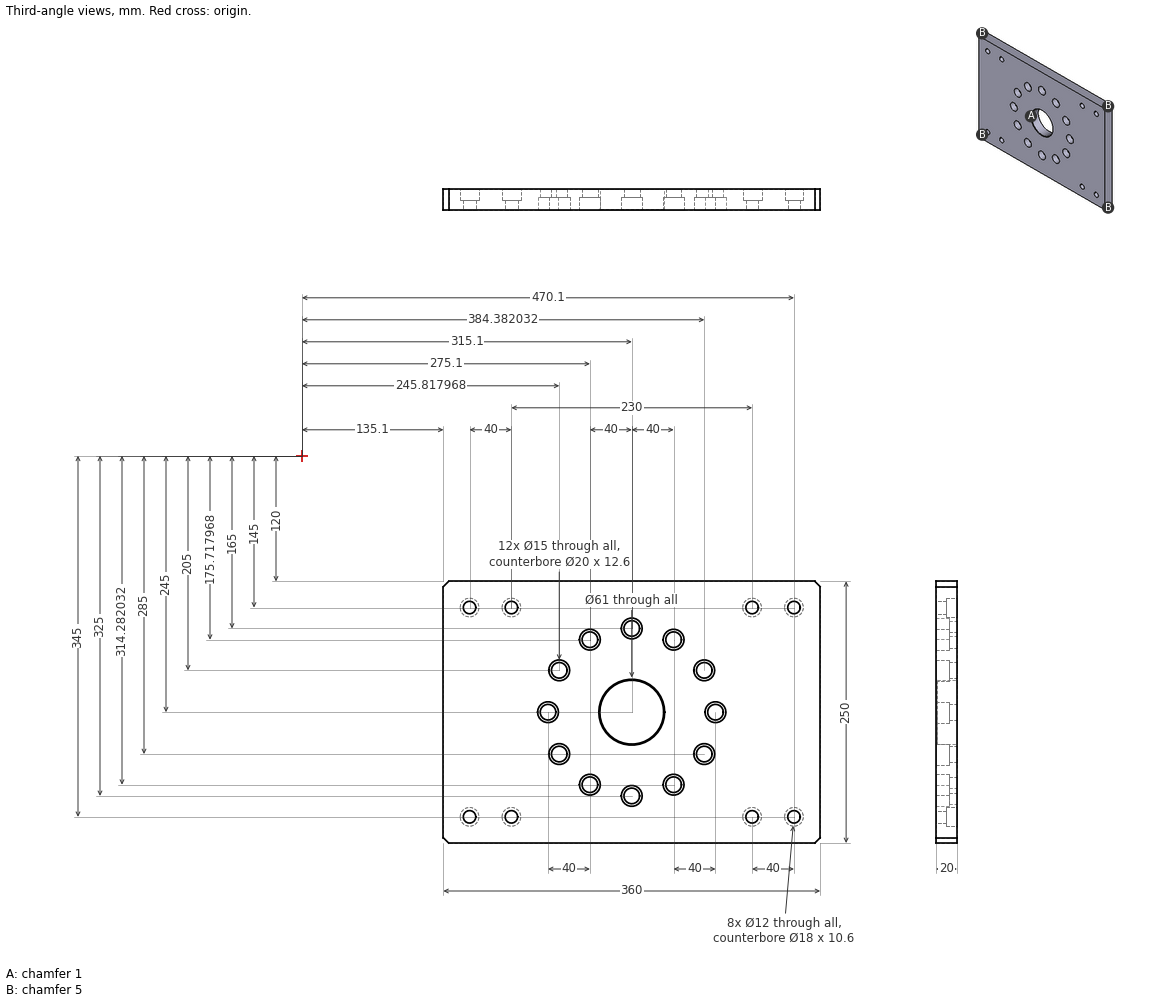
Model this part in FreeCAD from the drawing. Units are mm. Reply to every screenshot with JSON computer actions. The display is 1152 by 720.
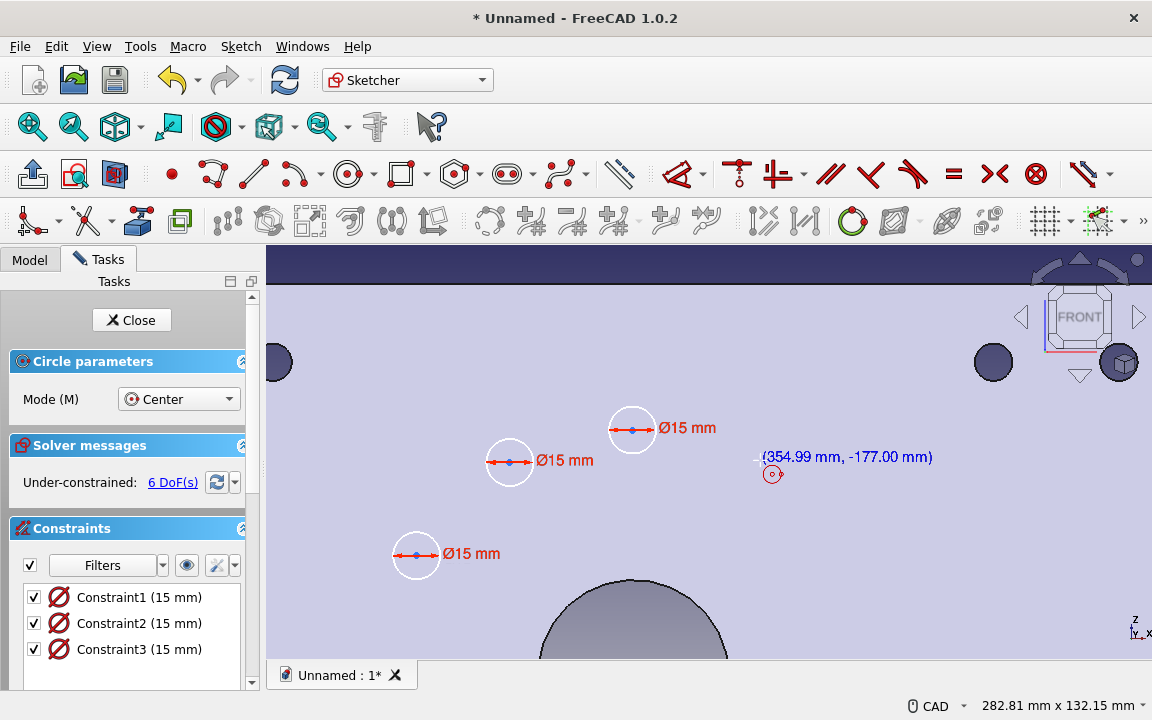
{"action": "scroll", "coordinate": [760, 460], "scroll_direction": "down", "scroll_amount": 7}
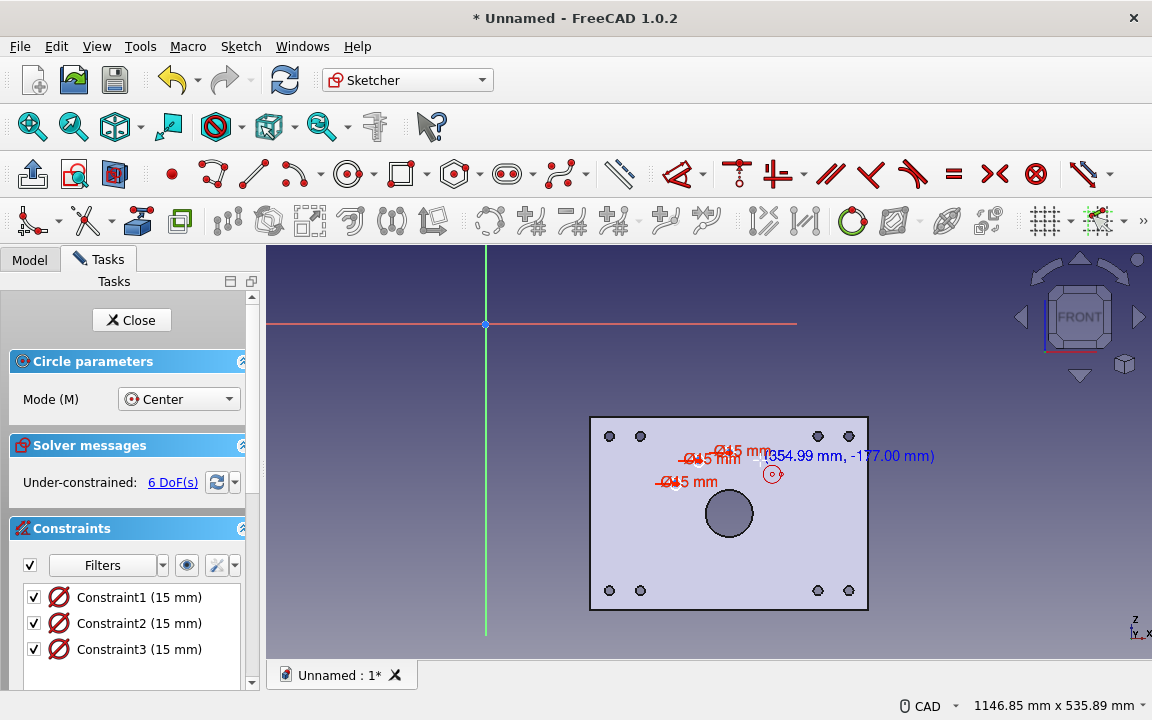
{"action": "left_click", "coordinate": [760, 460]}
{"action": "mouse_move", "coordinate": [764, 456]}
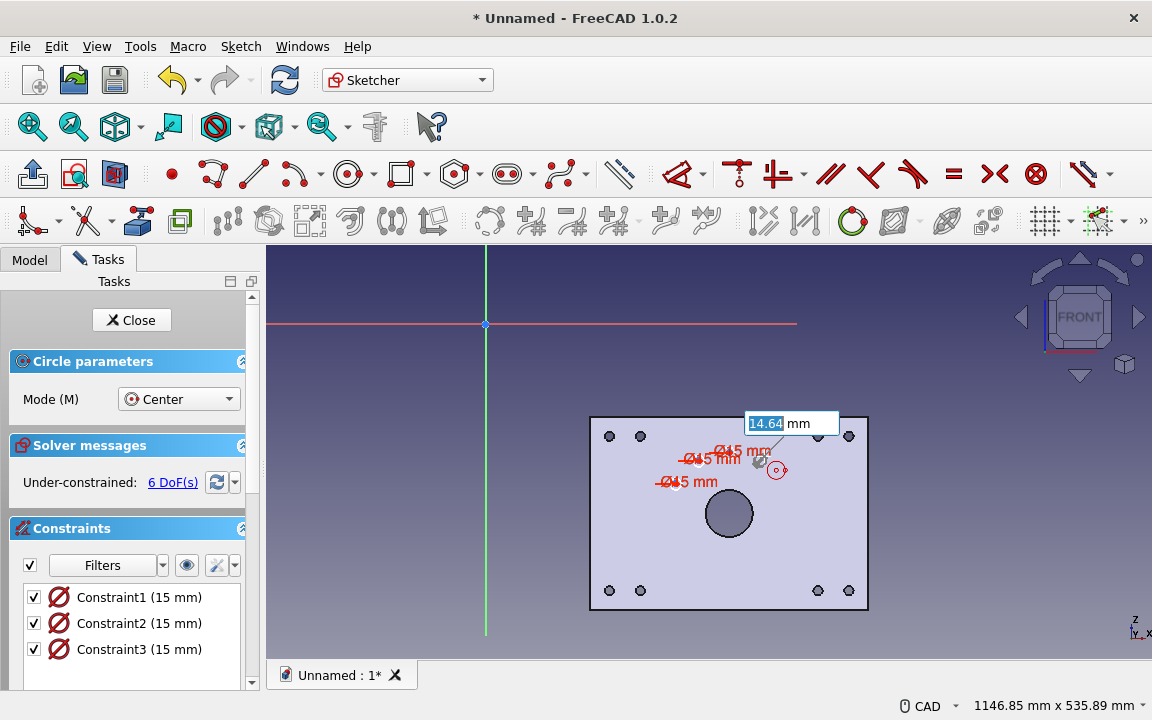
{"action": "type", "text": "15"}
{"action": "key", "text": "Return"}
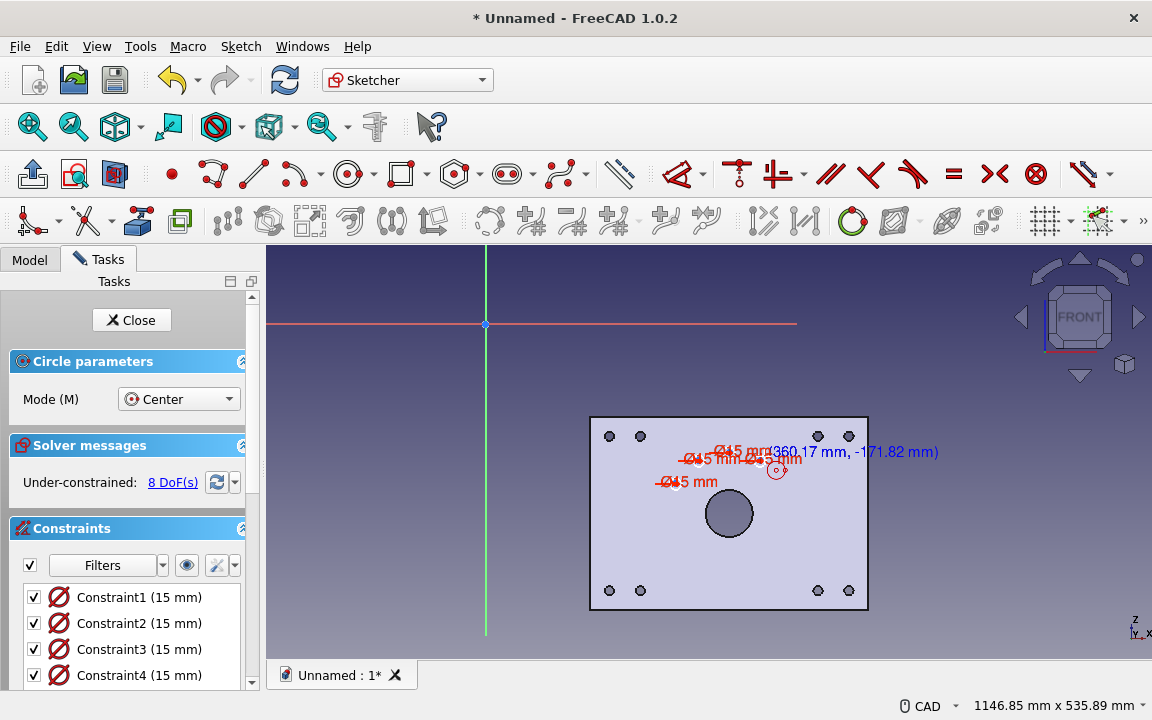
{"action": "scroll", "coordinate": [783, 483], "scroll_direction": "up", "scroll_amount": 7}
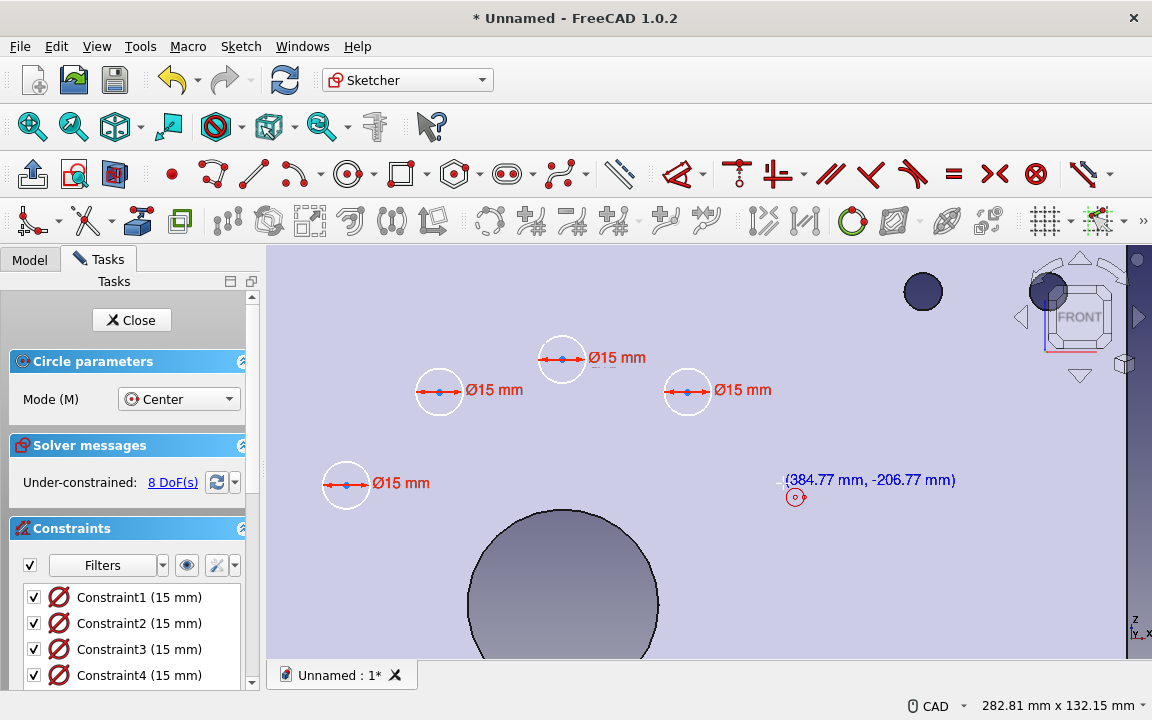
{"action": "scroll", "coordinate": [783, 483], "scroll_direction": "down", "scroll_amount": 7}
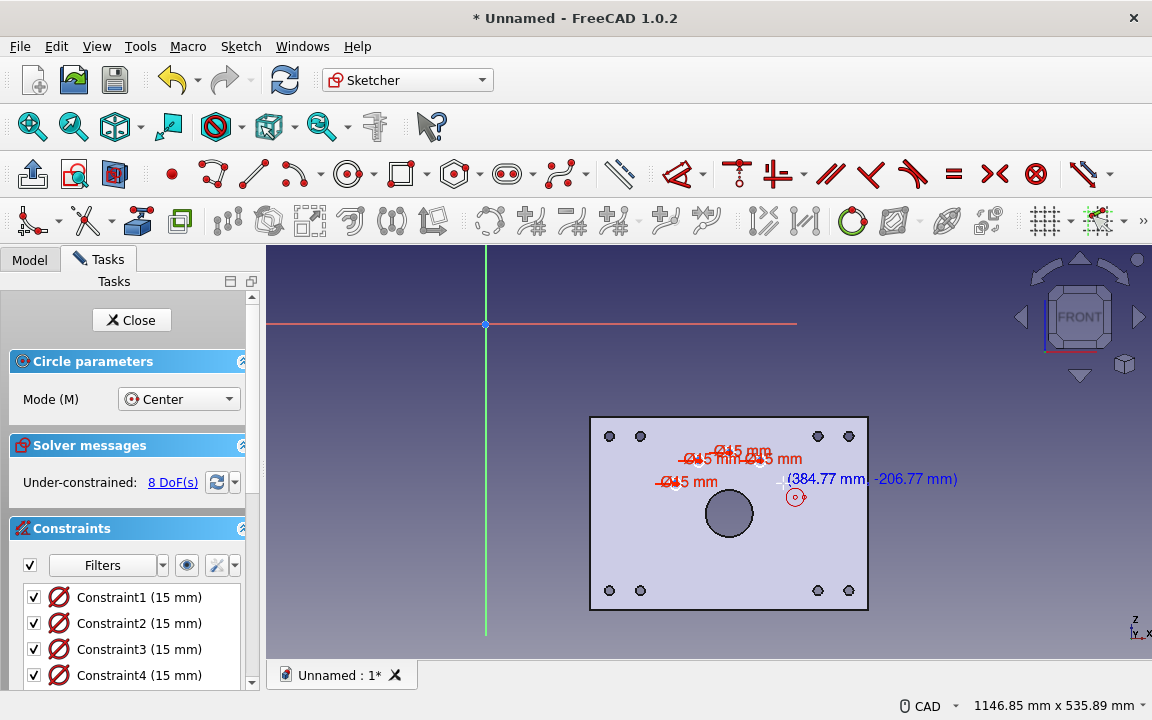
{"action": "left_click", "coordinate": [783, 483]}
{"action": "mouse_move", "coordinate": [787, 479]}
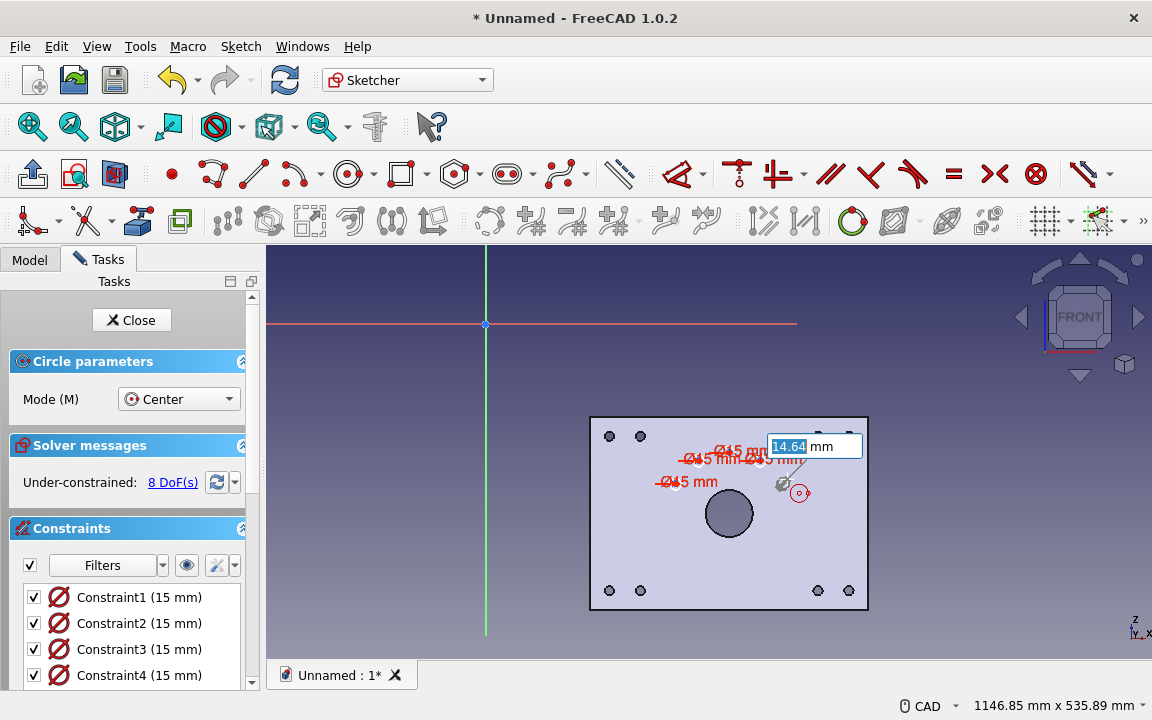
{"action": "type", "text": "15"}
{"action": "key", "text": "Return"}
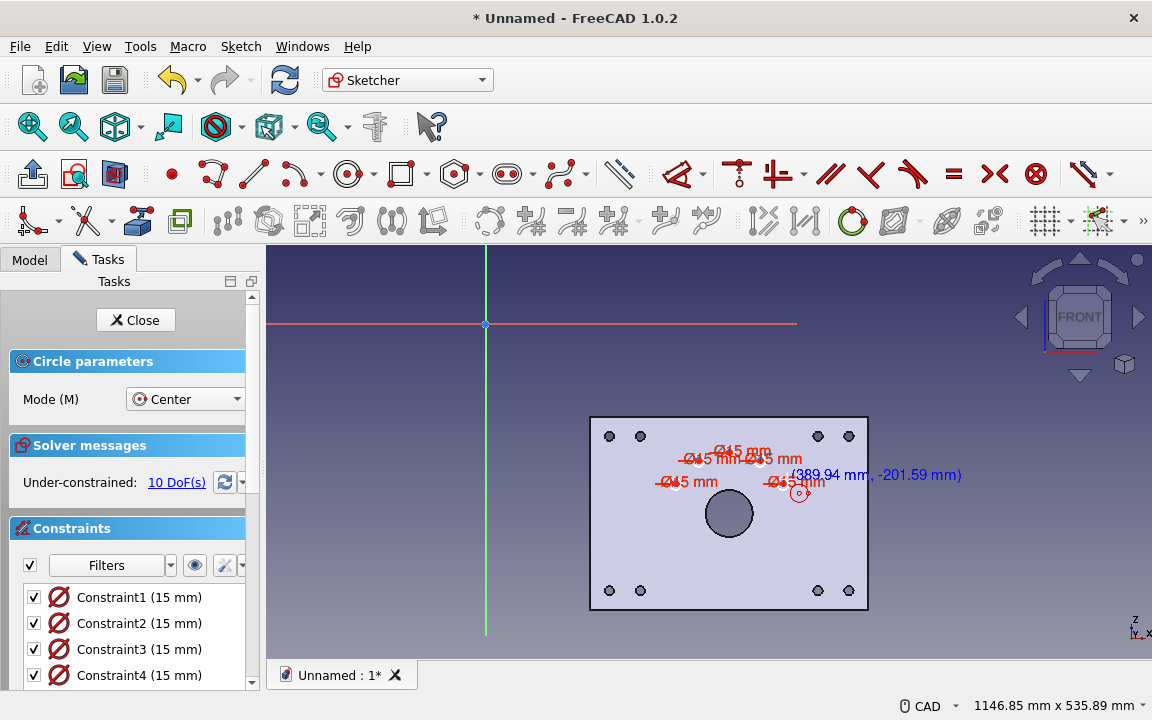
{"action": "scroll", "coordinate": [791, 514], "scroll_direction": "up", "scroll_amount": 7}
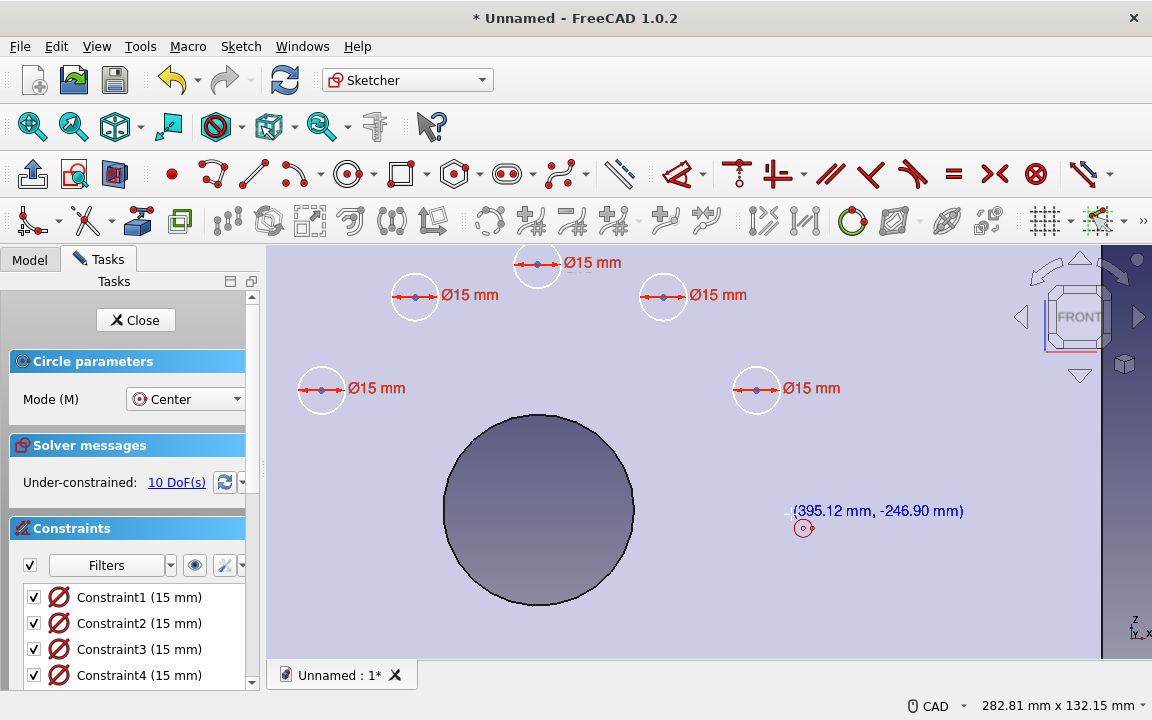
{"action": "scroll", "coordinate": [791, 514], "scroll_direction": "down", "scroll_amount": 7}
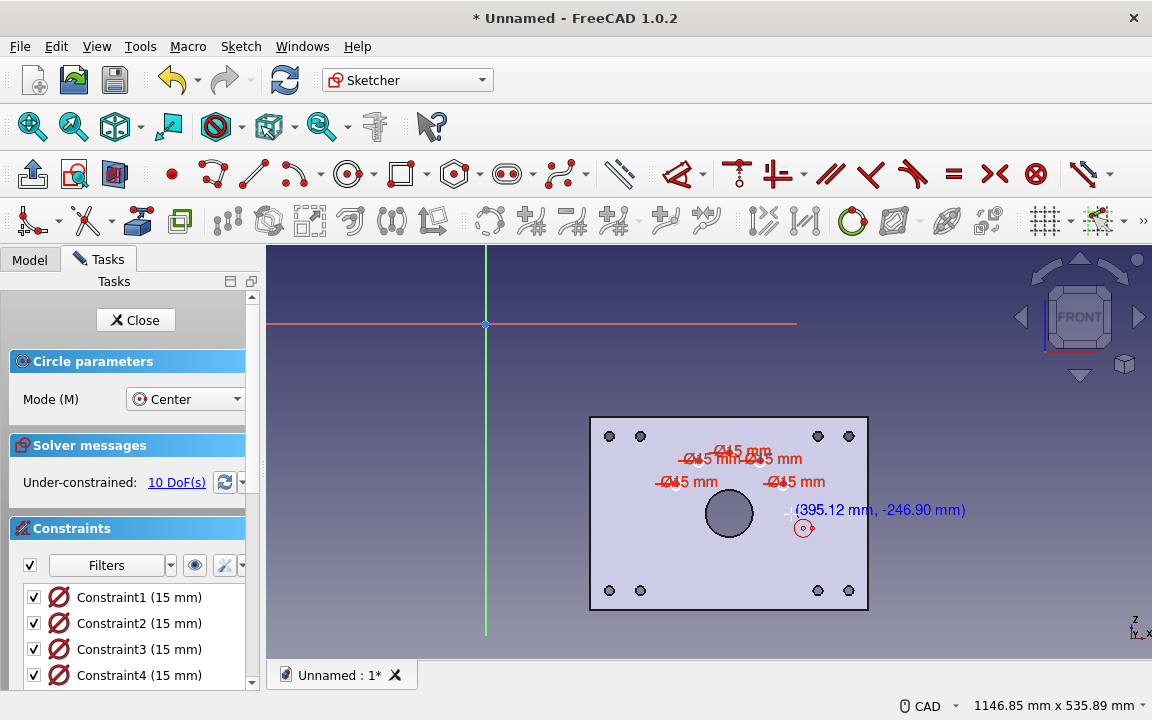
{"action": "left_click", "coordinate": [791, 514]}
{"action": "mouse_move", "coordinate": [795, 509]}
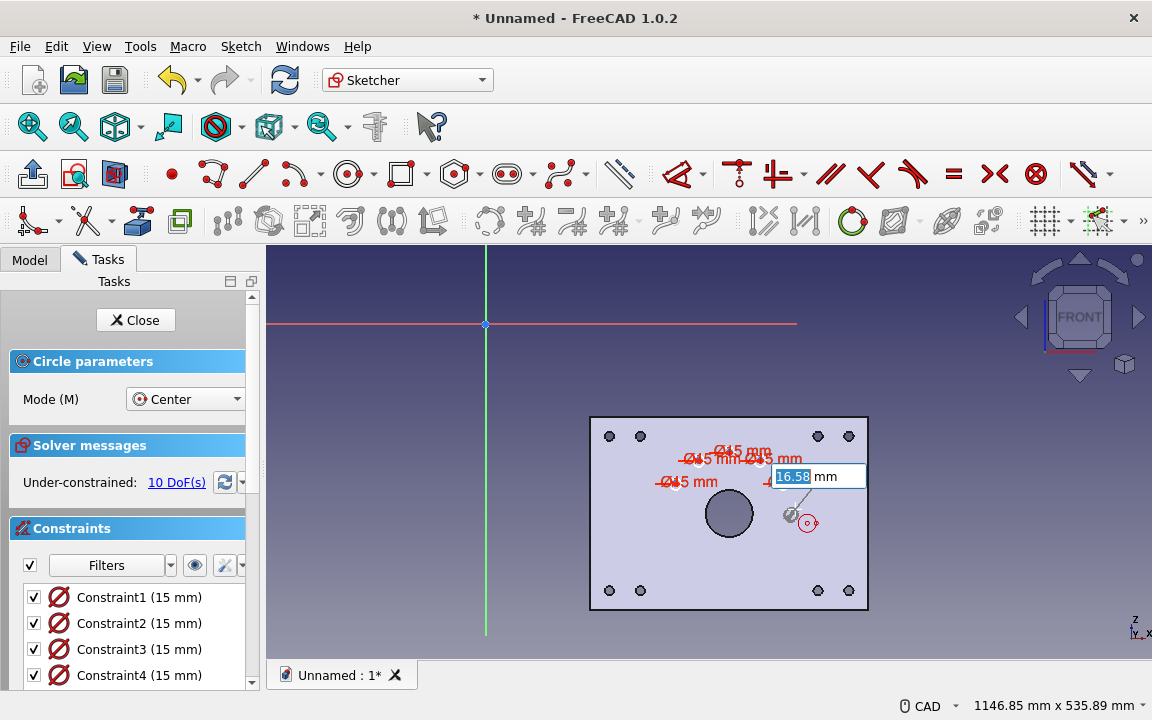
{"action": "type", "text": "15"}
{"action": "key", "text": "Return"}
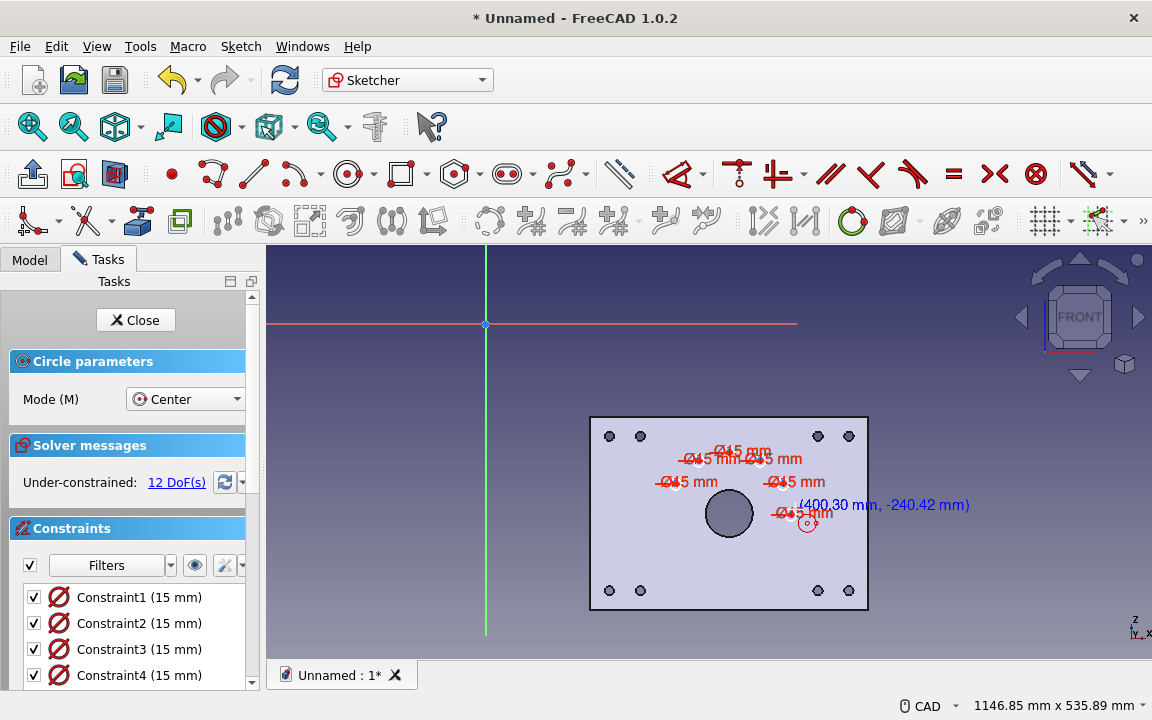
{"action": "scroll", "coordinate": [783, 544], "scroll_direction": "up", "scroll_amount": 7}